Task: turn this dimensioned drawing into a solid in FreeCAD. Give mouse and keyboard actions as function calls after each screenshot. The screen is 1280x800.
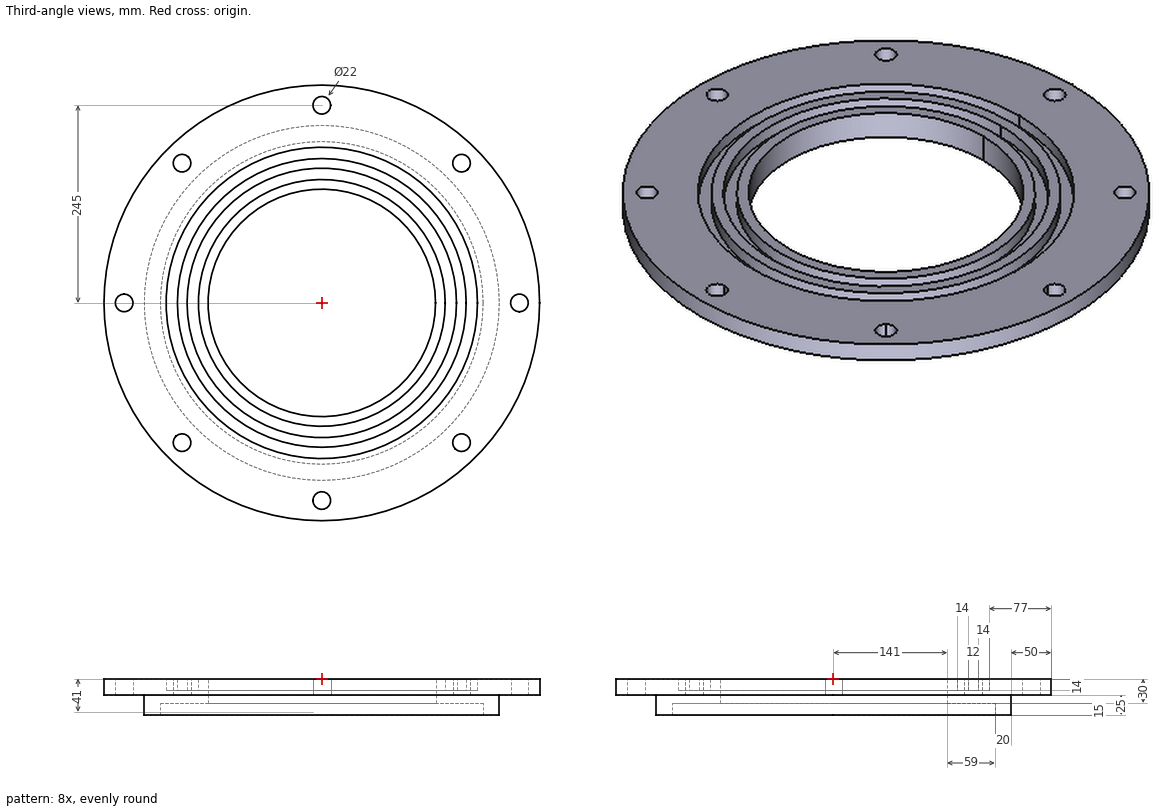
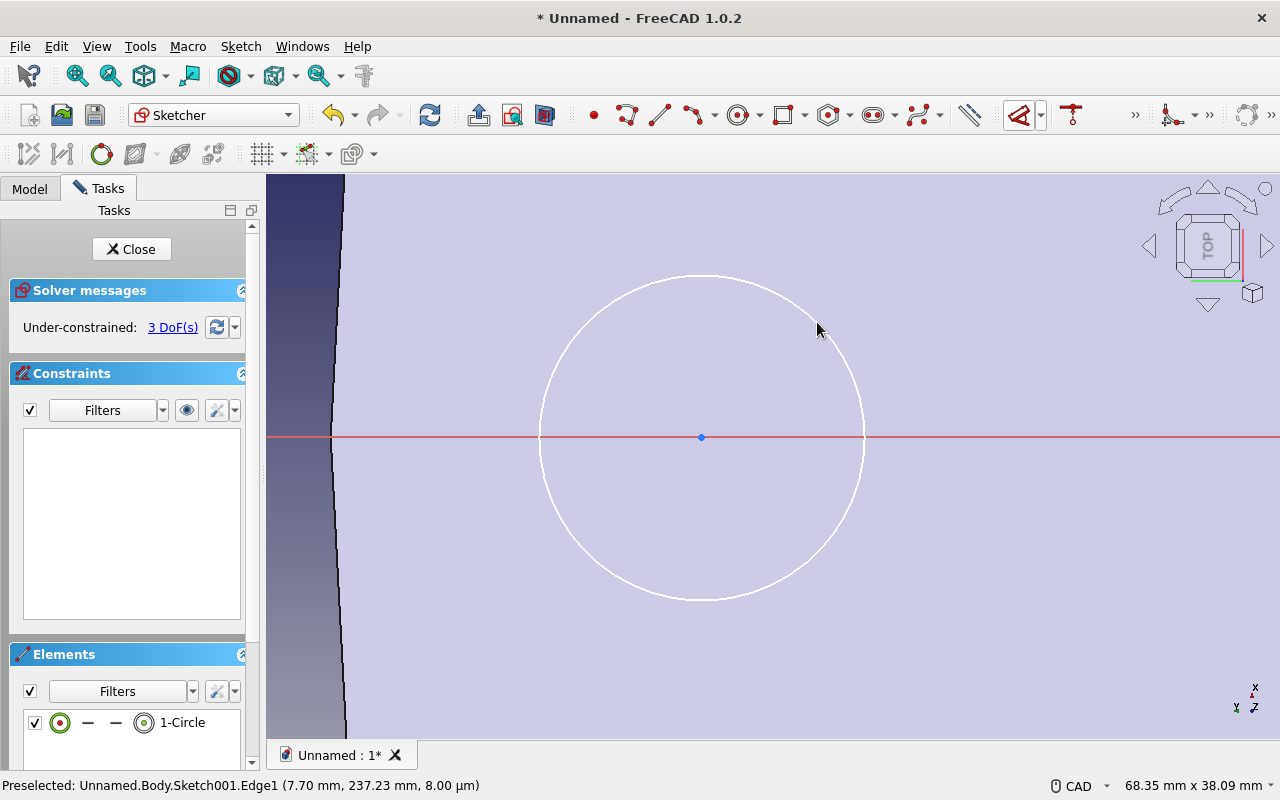
click(702, 438)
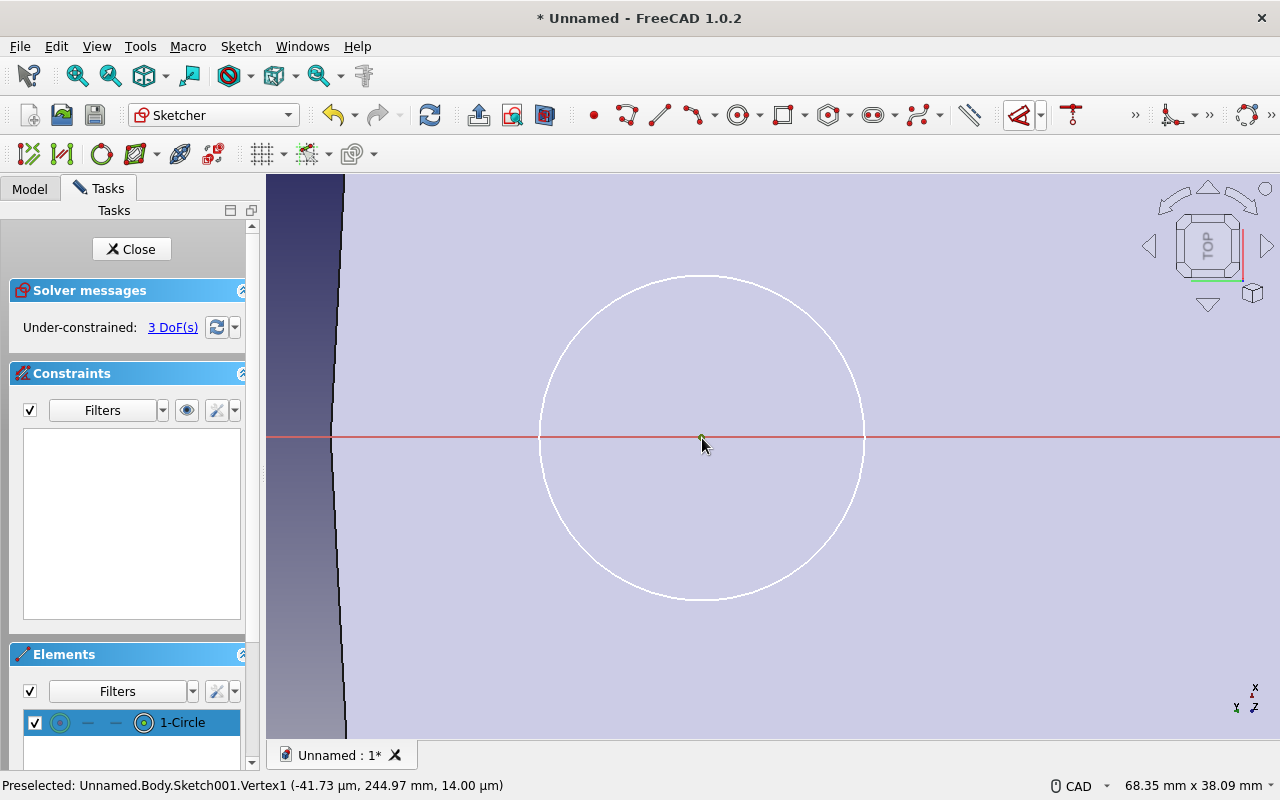
click(353, 437)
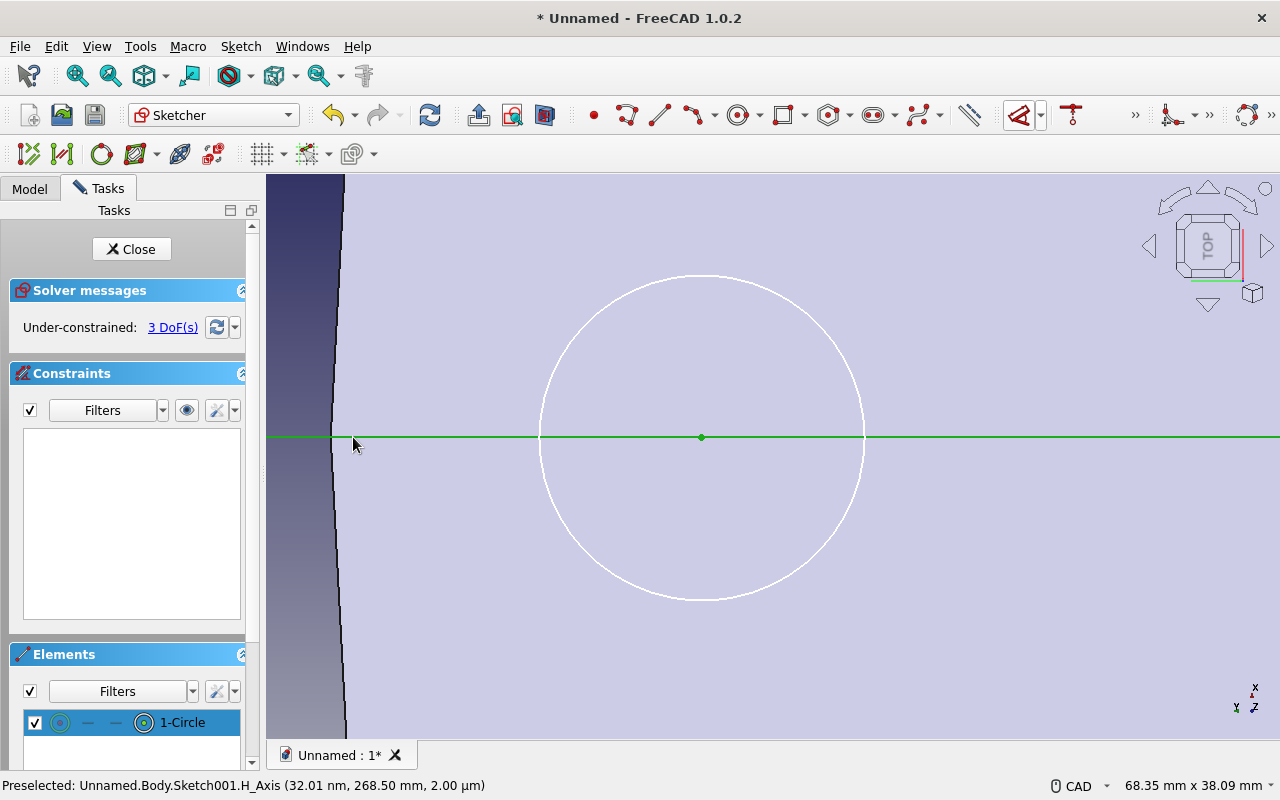
click(1071, 116)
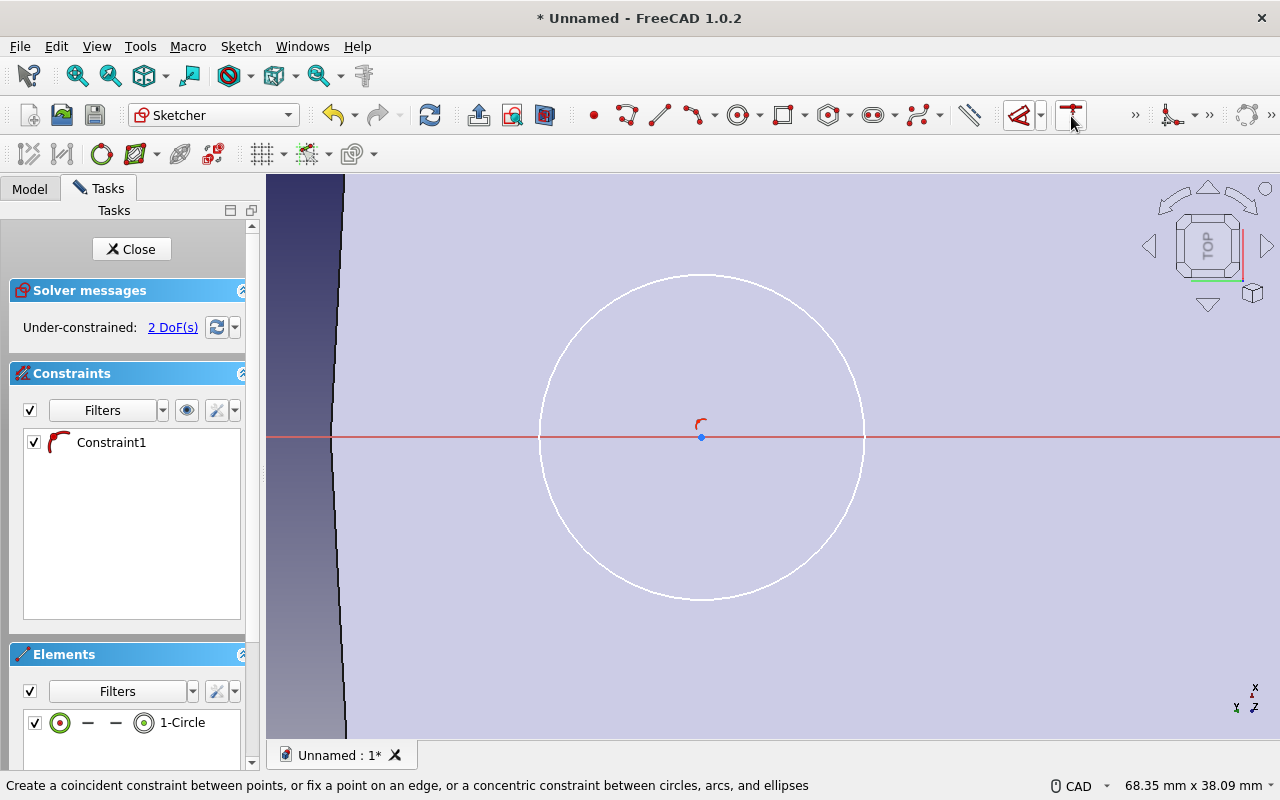
click(817, 322)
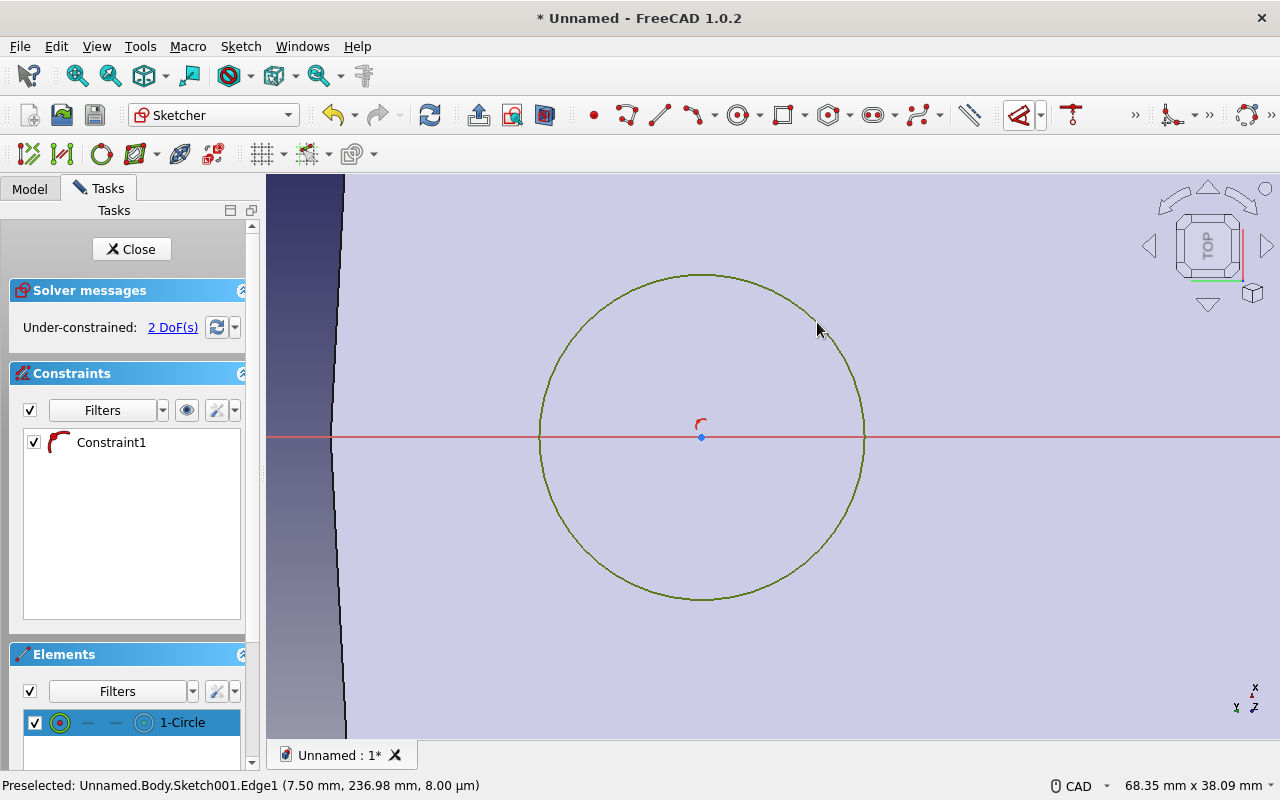
click(1040, 116)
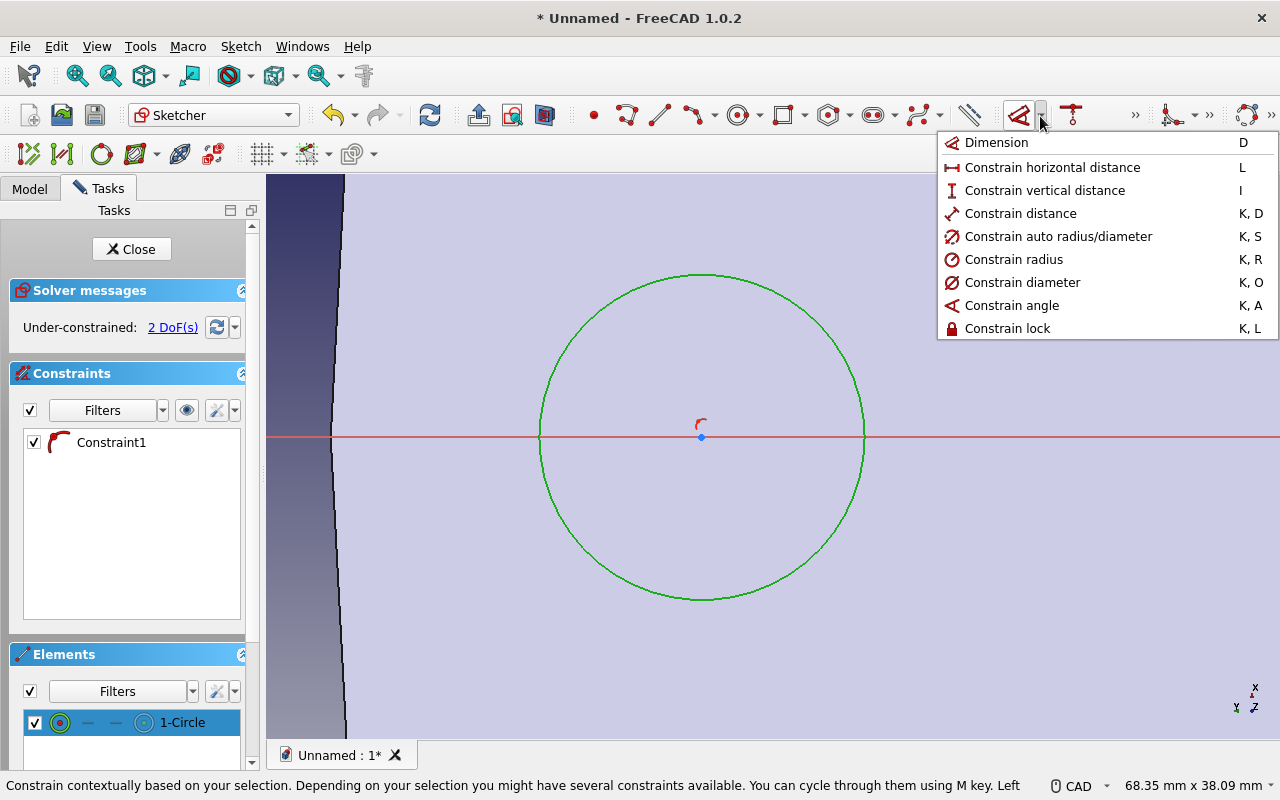
click(1108, 282)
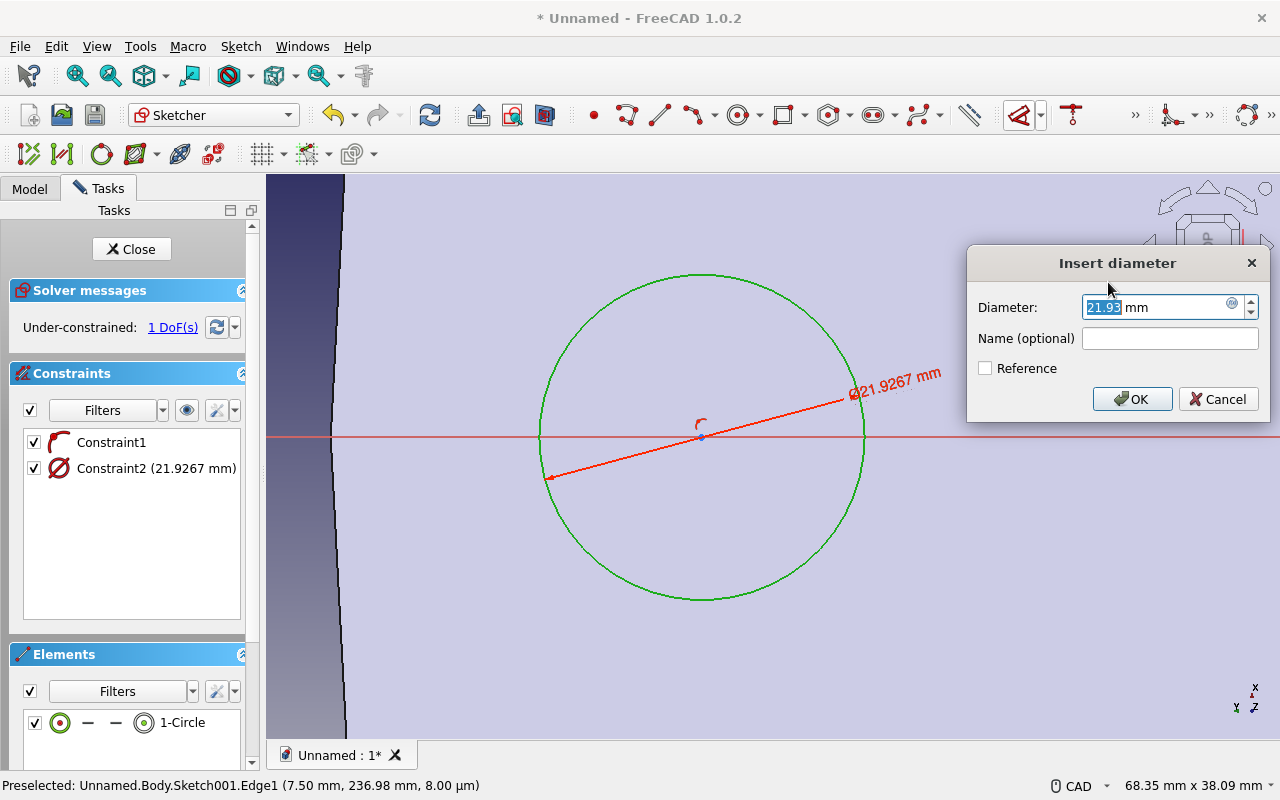
text(22)
key(Return)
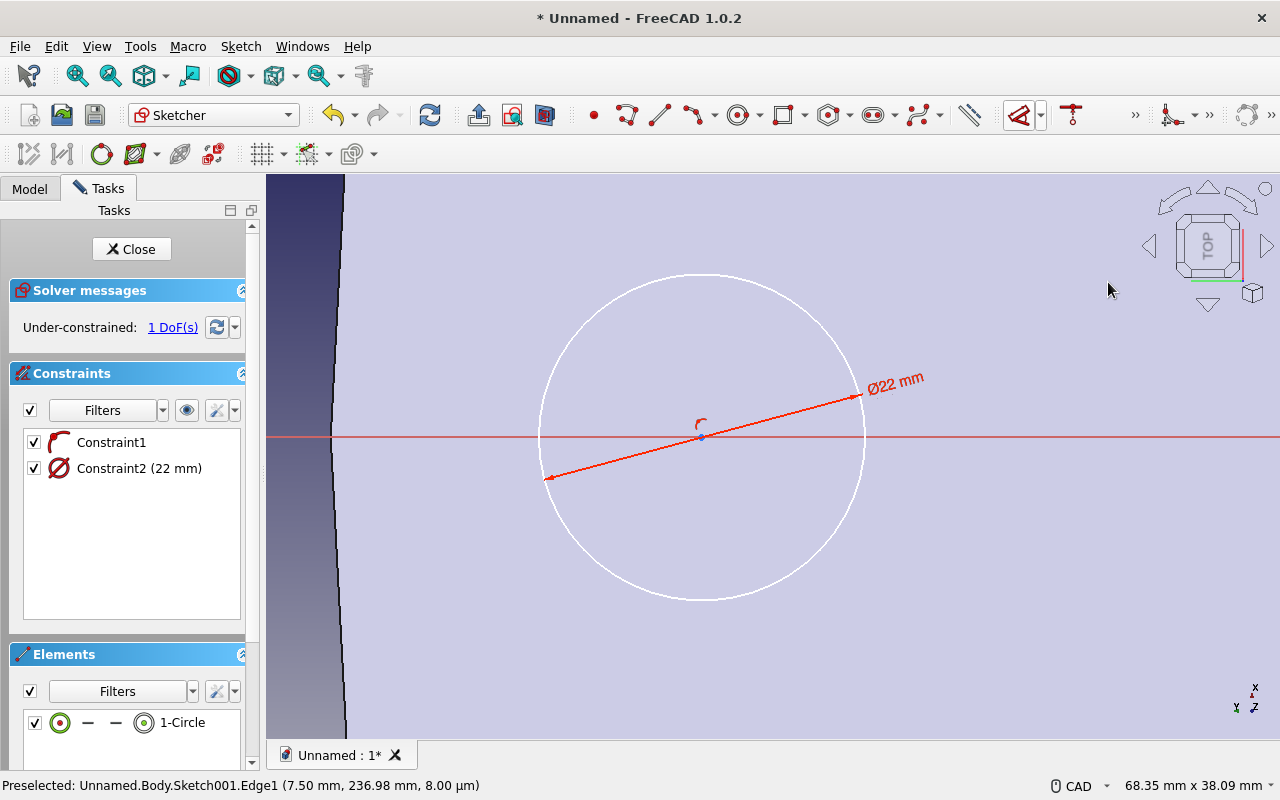
click(702, 437)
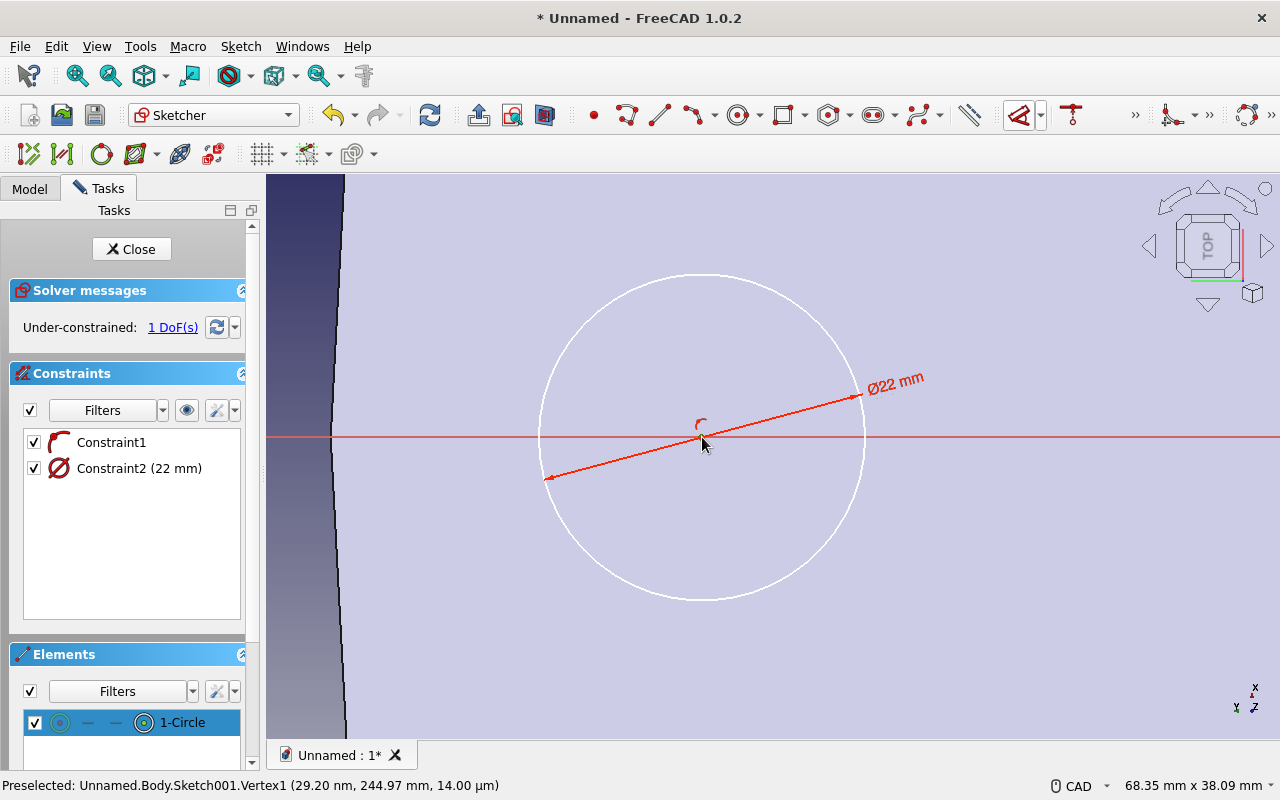
click(1040, 116)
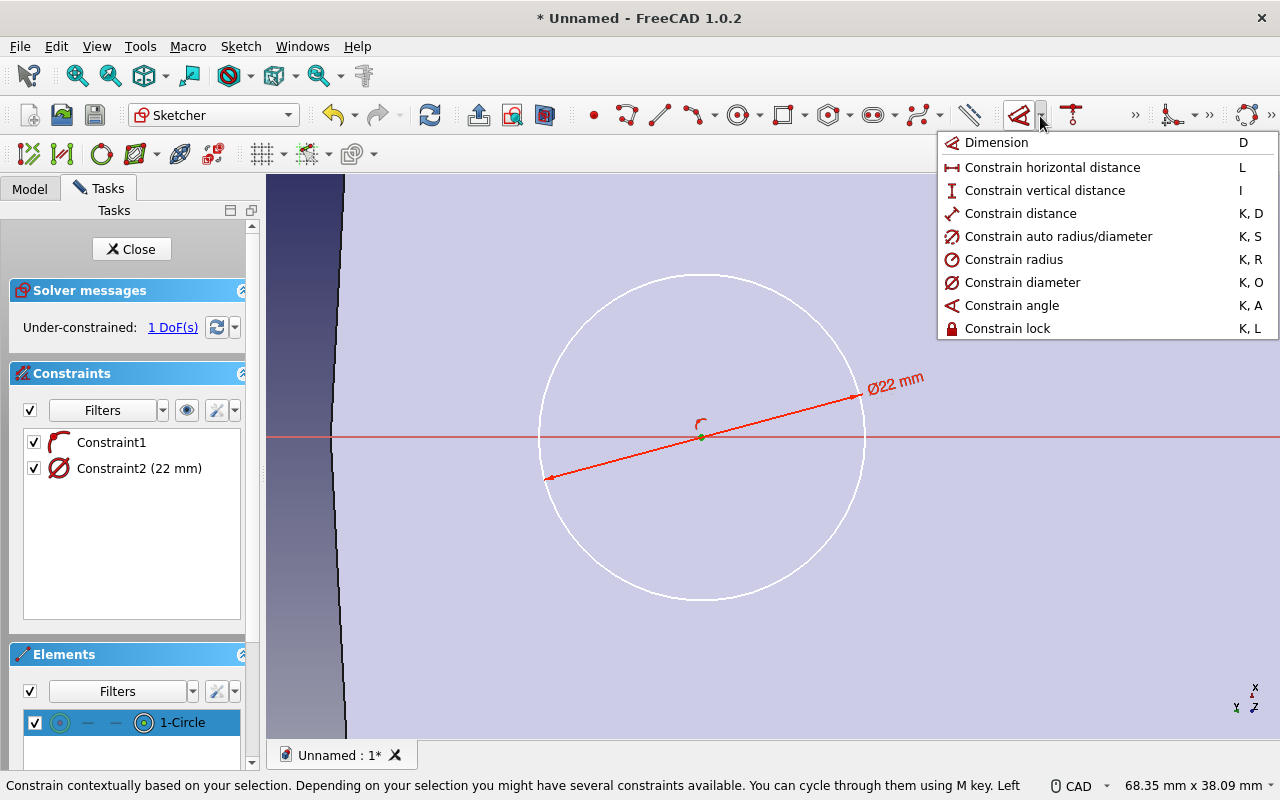
click(1108, 168)